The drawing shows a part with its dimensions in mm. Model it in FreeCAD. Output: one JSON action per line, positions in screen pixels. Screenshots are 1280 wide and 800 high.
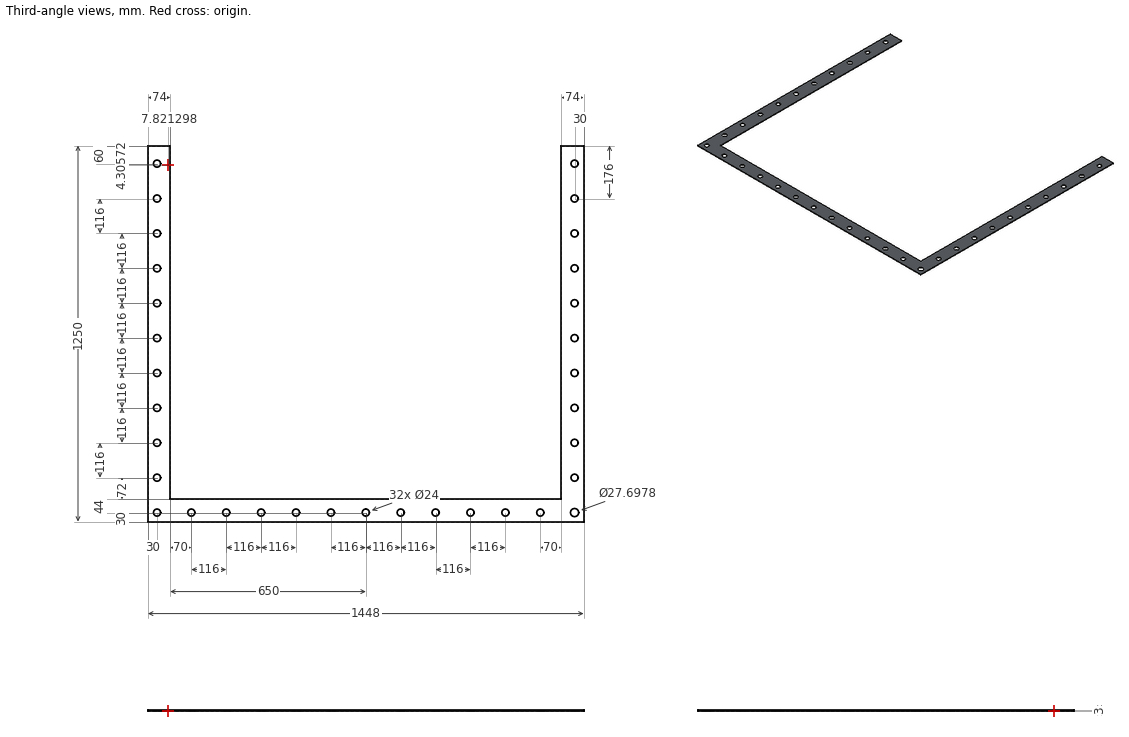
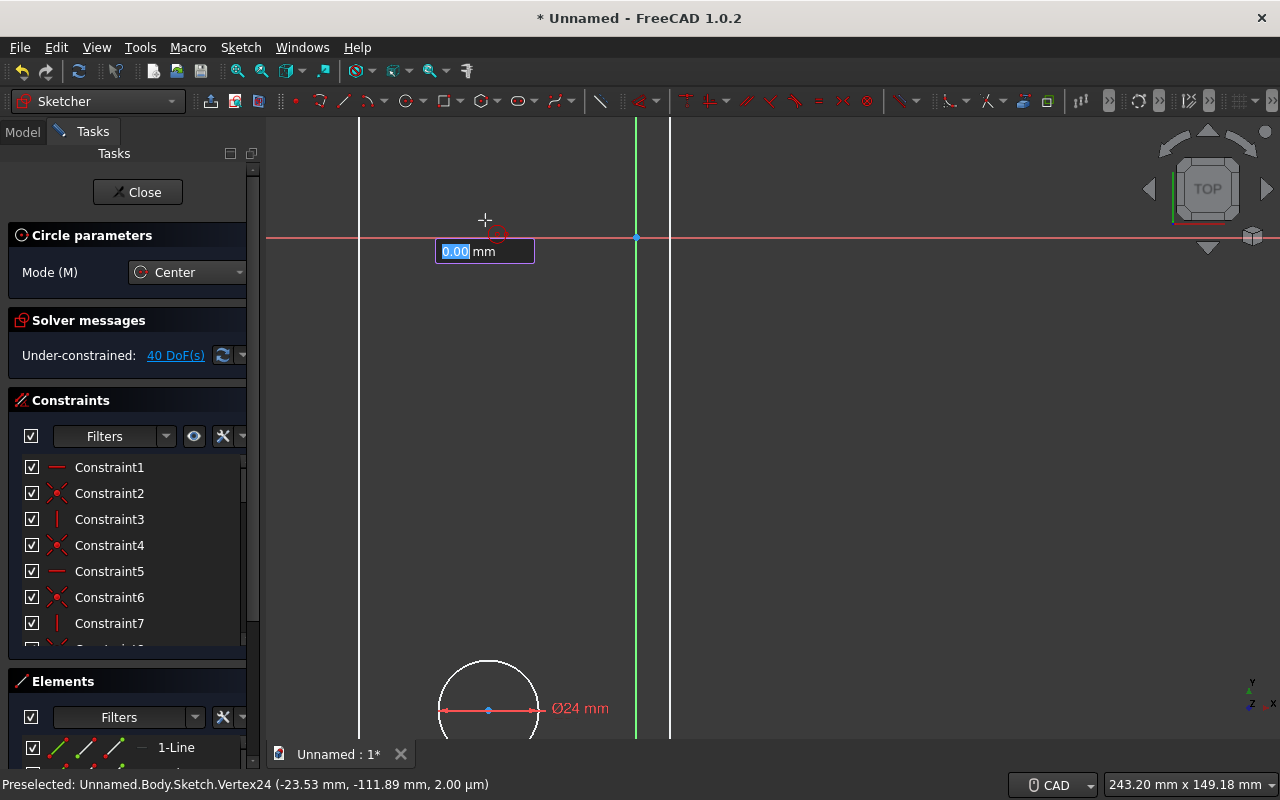
{"action": "scroll", "coordinate": [490, 256], "scroll_direction": "down", "scroll_amount": 13}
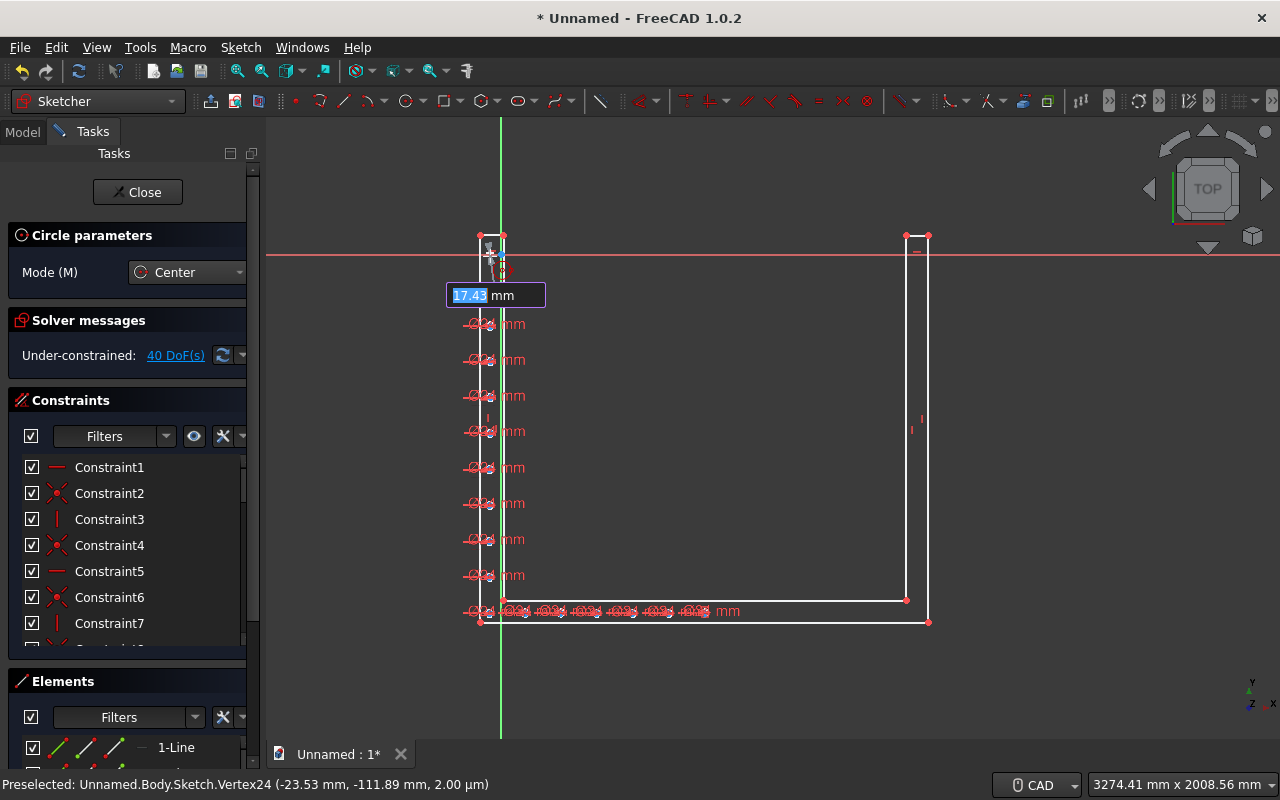
{"action": "scroll", "coordinate": [492, 251], "scroll_direction": "up", "scroll_amount": 7}
{"action": "mouse_move", "coordinate": [493, 250]}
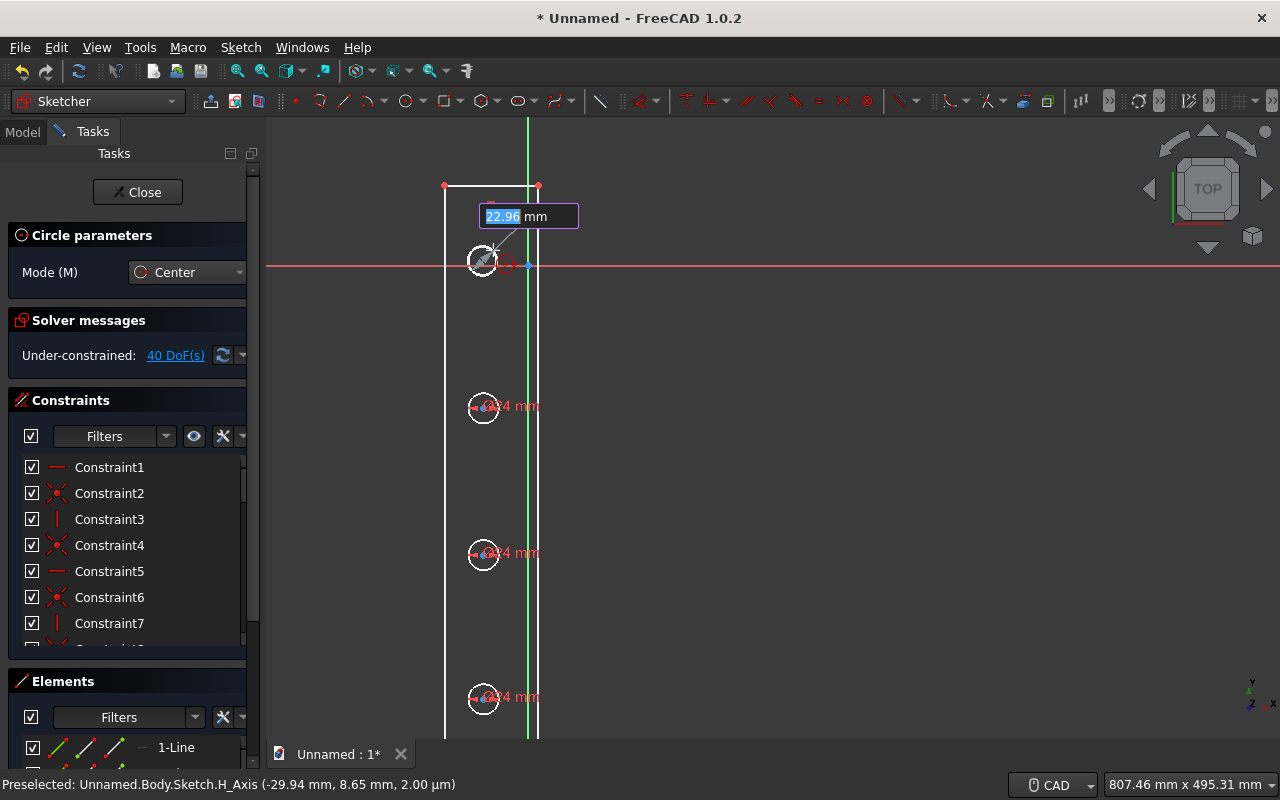
{"action": "type", "text": "24"}
{"action": "key", "text": "Return"}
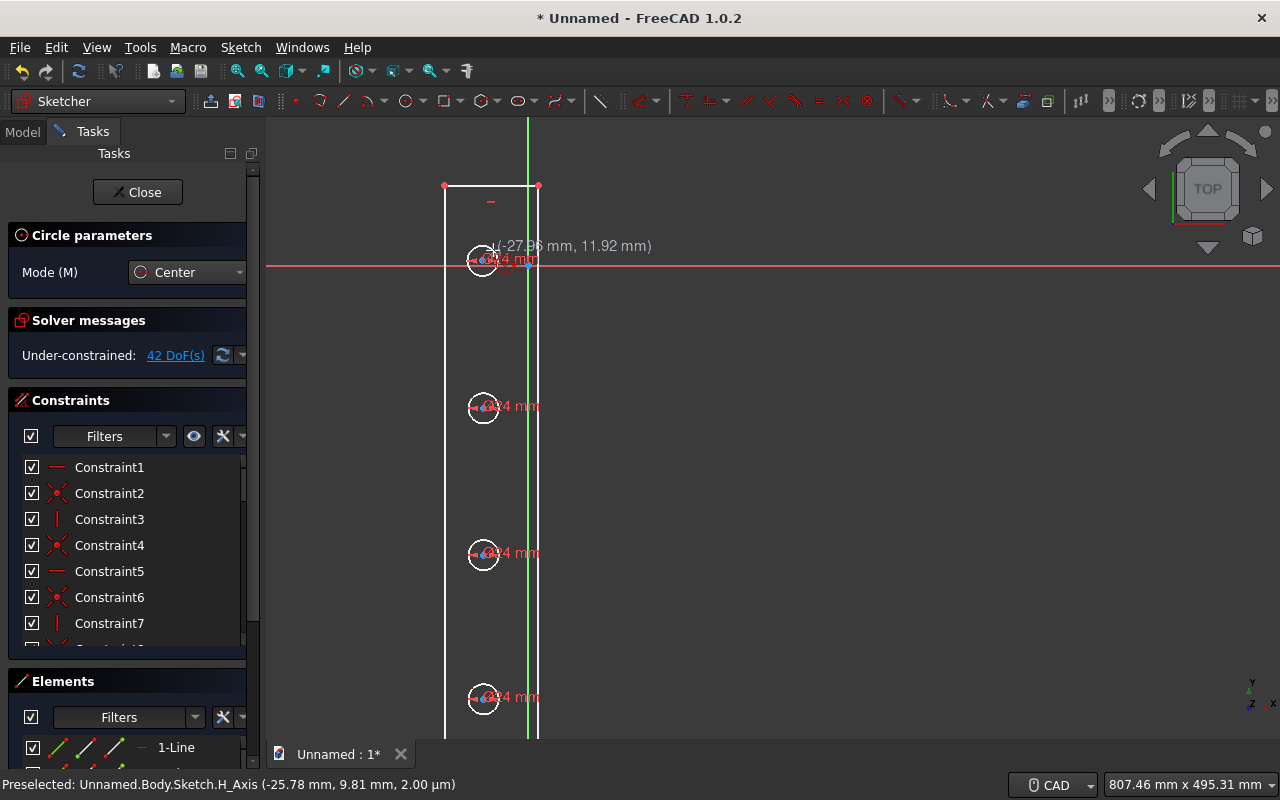
{"action": "scroll", "coordinate": [492, 251], "scroll_direction": "down", "scroll_amount": 7}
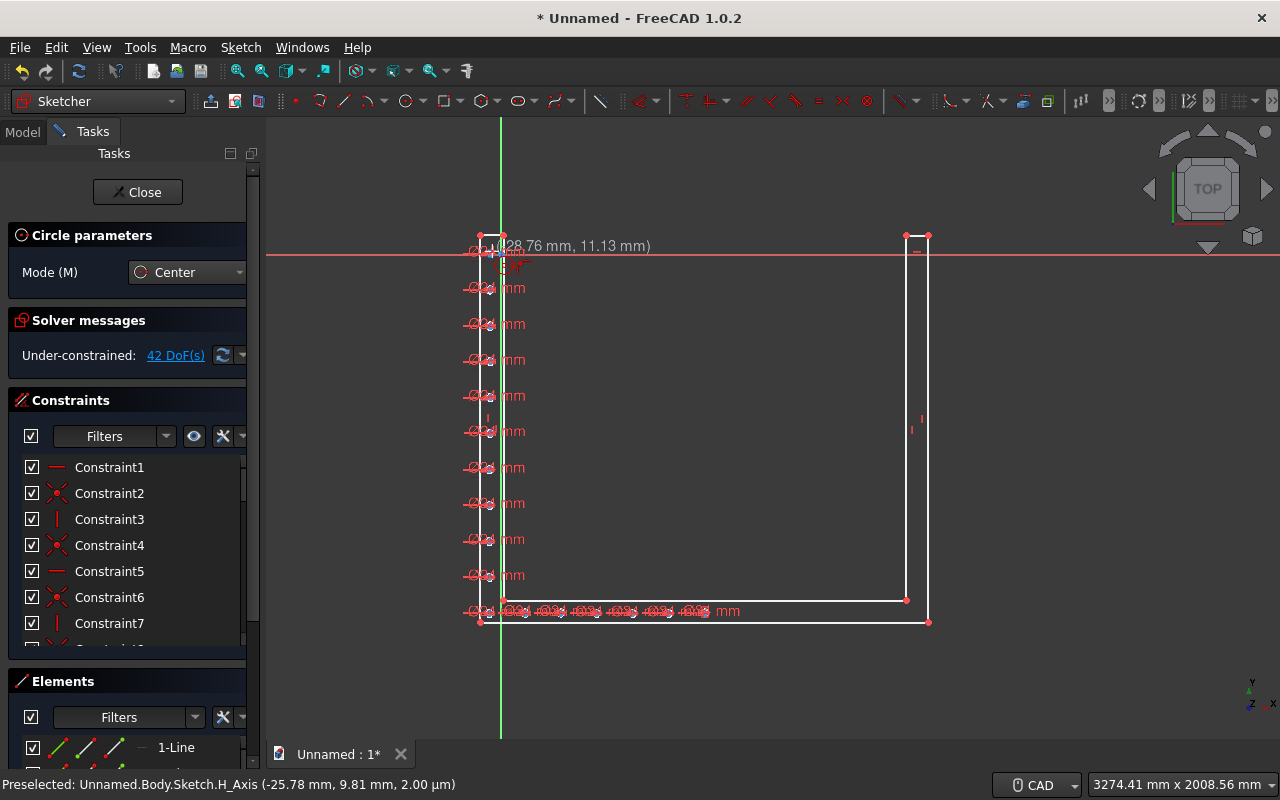
{"action": "scroll", "coordinate": [920, 289], "scroll_direction": "up", "scroll_amount": 10}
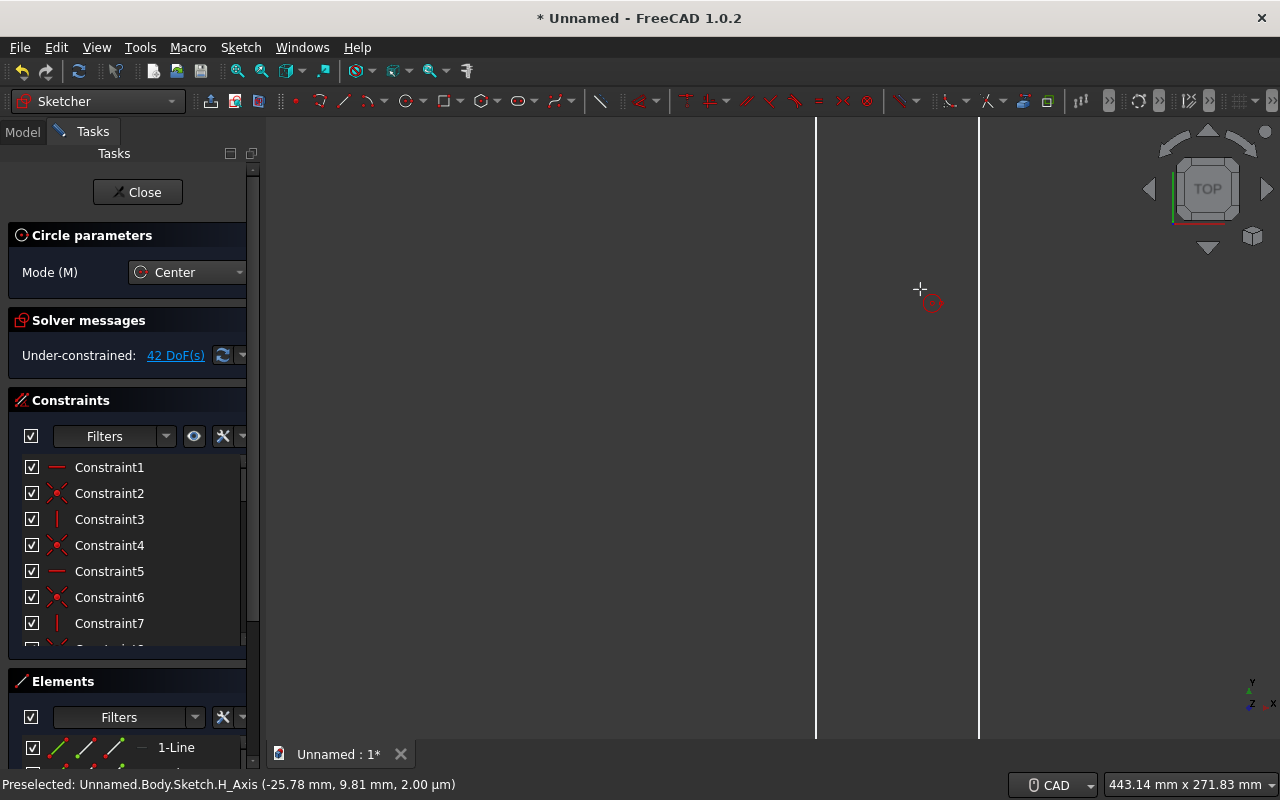
{"action": "scroll", "coordinate": [920, 289], "scroll_direction": "down", "scroll_amount": 10}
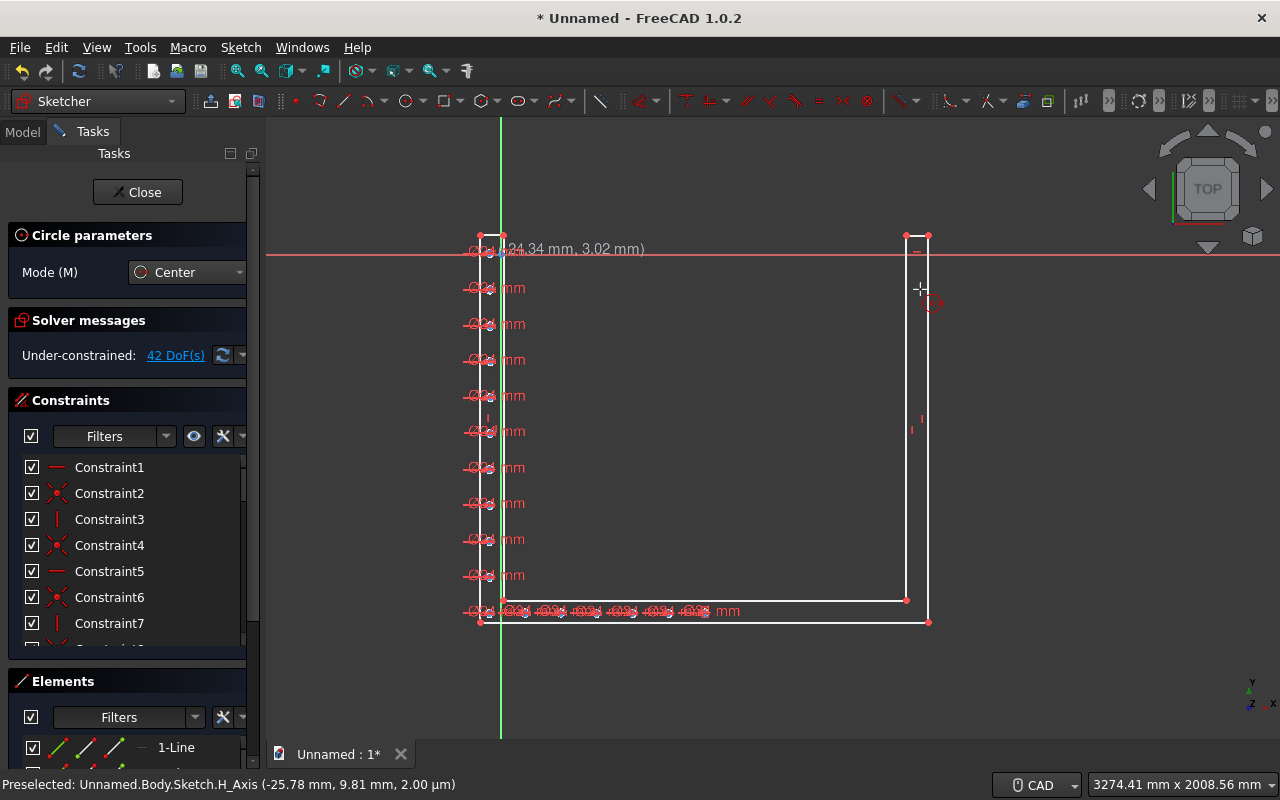
{"action": "scroll", "coordinate": [920, 289], "scroll_direction": "up", "scroll_amount": 3}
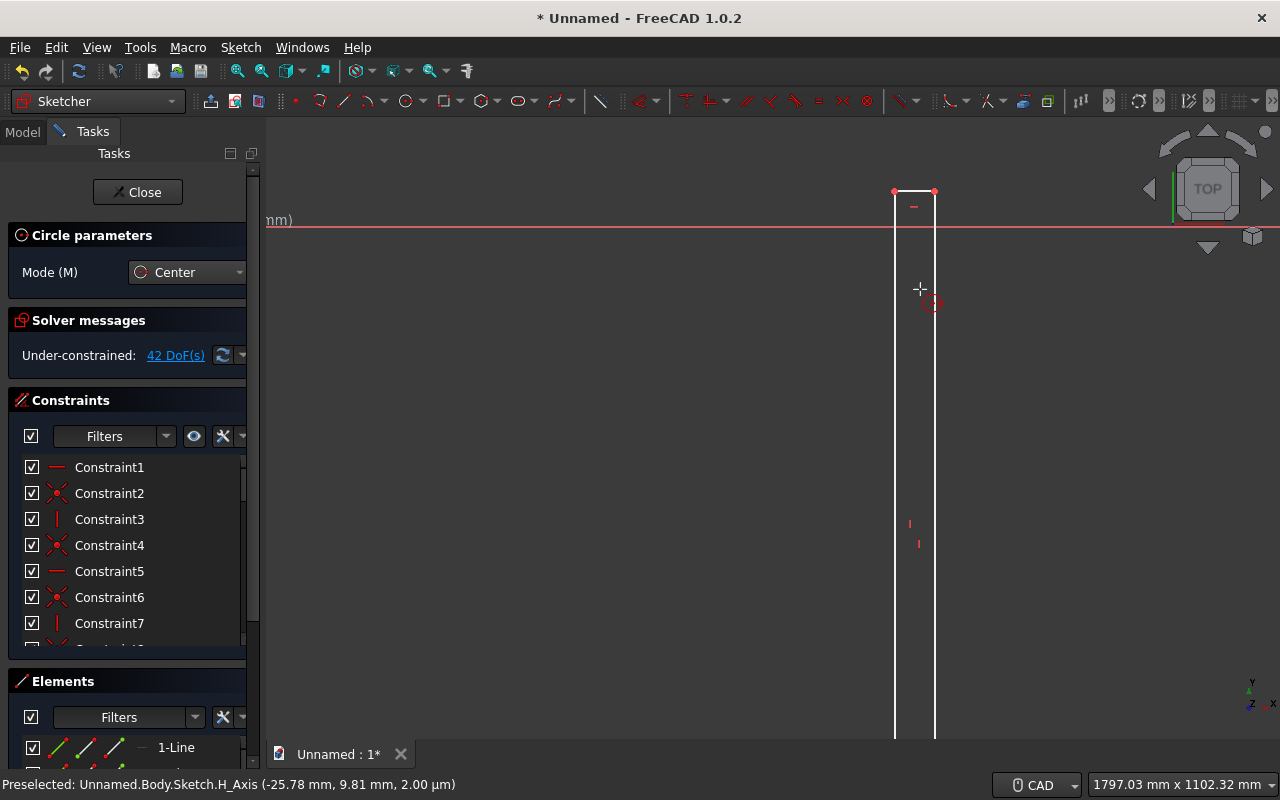
{"action": "left_click", "coordinate": [919, 290]}
{"action": "mouse_move", "coordinate": [914, 285]}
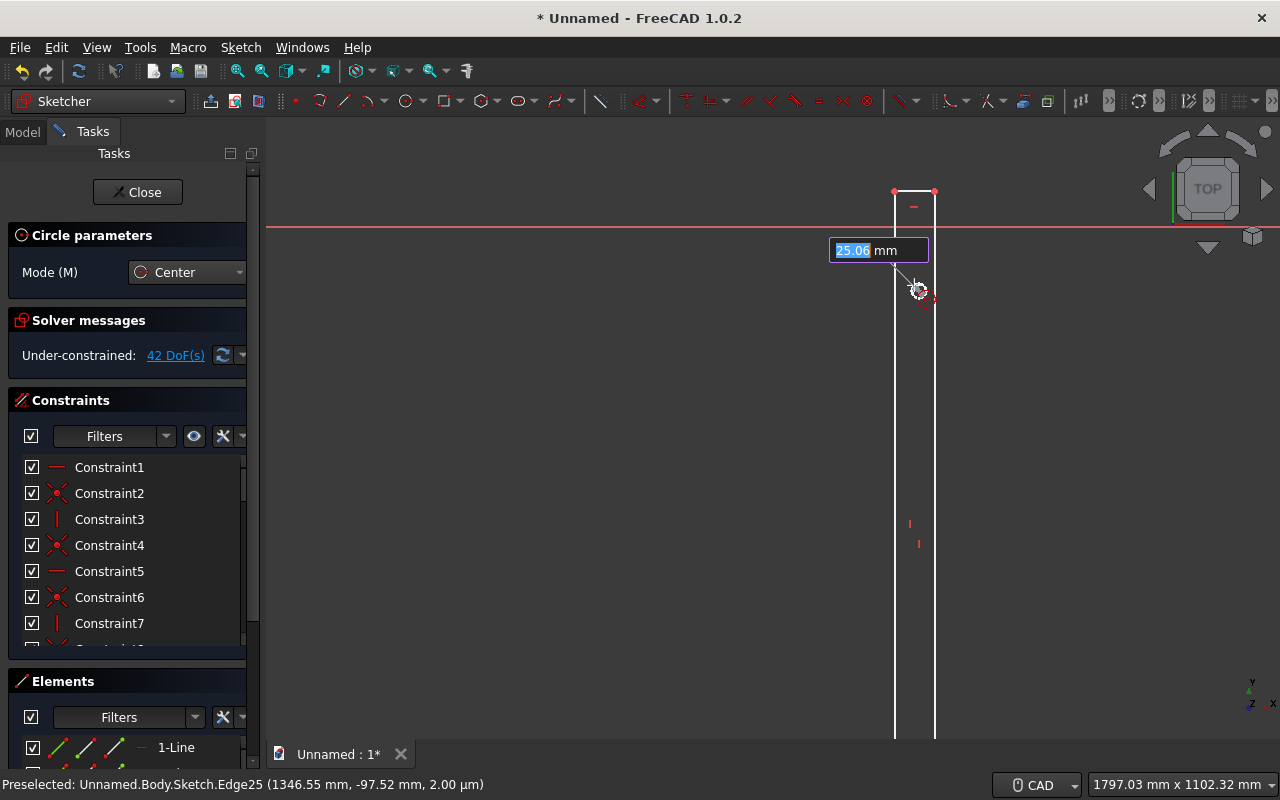
{"action": "type", "text": "24"}
{"action": "key", "text": "Return"}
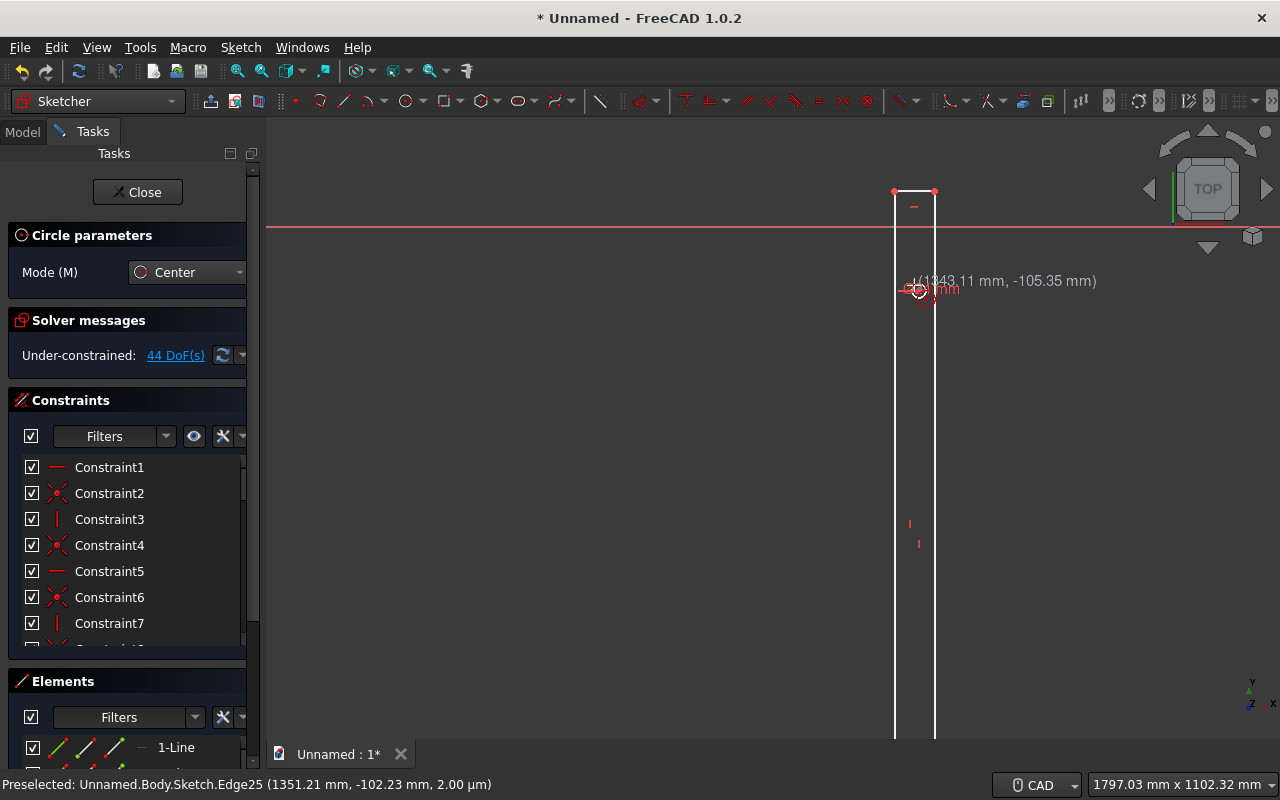
{"action": "scroll", "coordinate": [919, 224], "scroll_direction": "up", "scroll_amount": 10}